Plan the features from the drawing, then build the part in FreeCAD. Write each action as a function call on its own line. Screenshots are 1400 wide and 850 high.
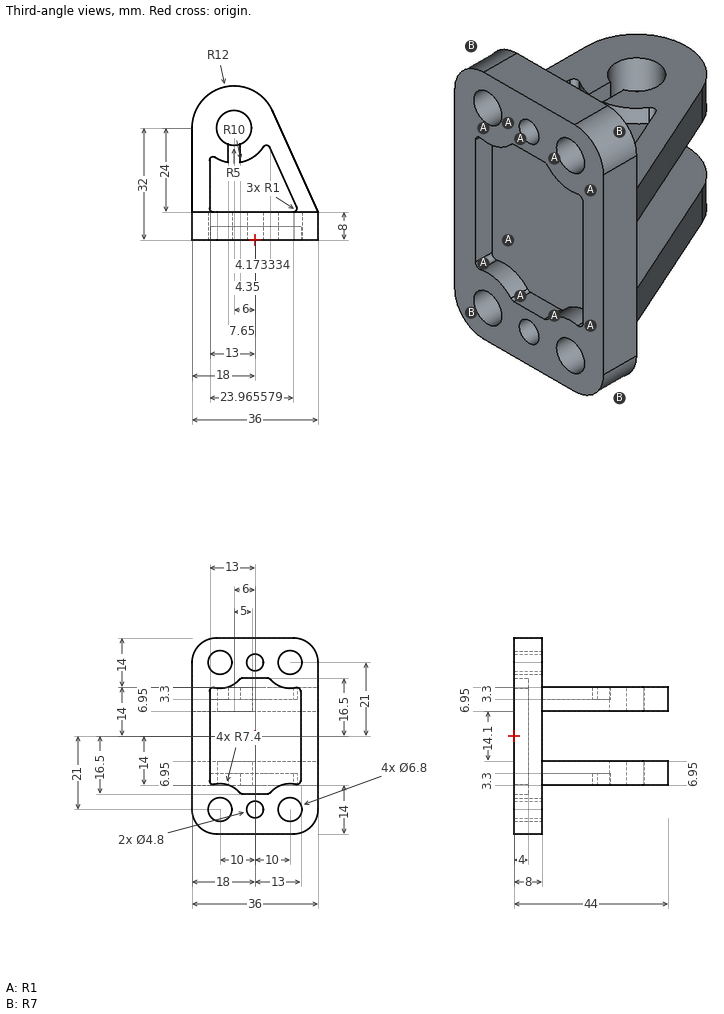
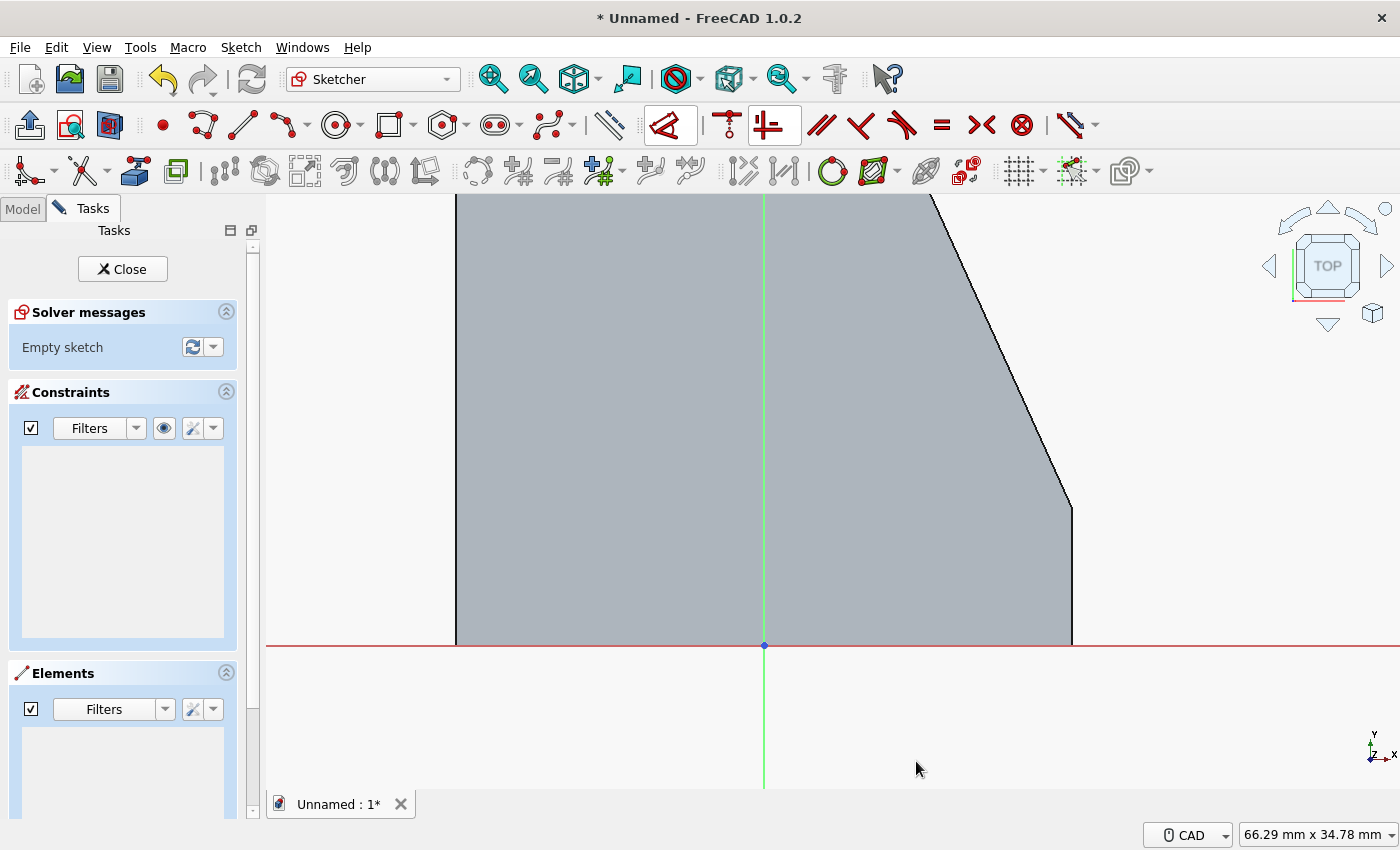
click(390, 126)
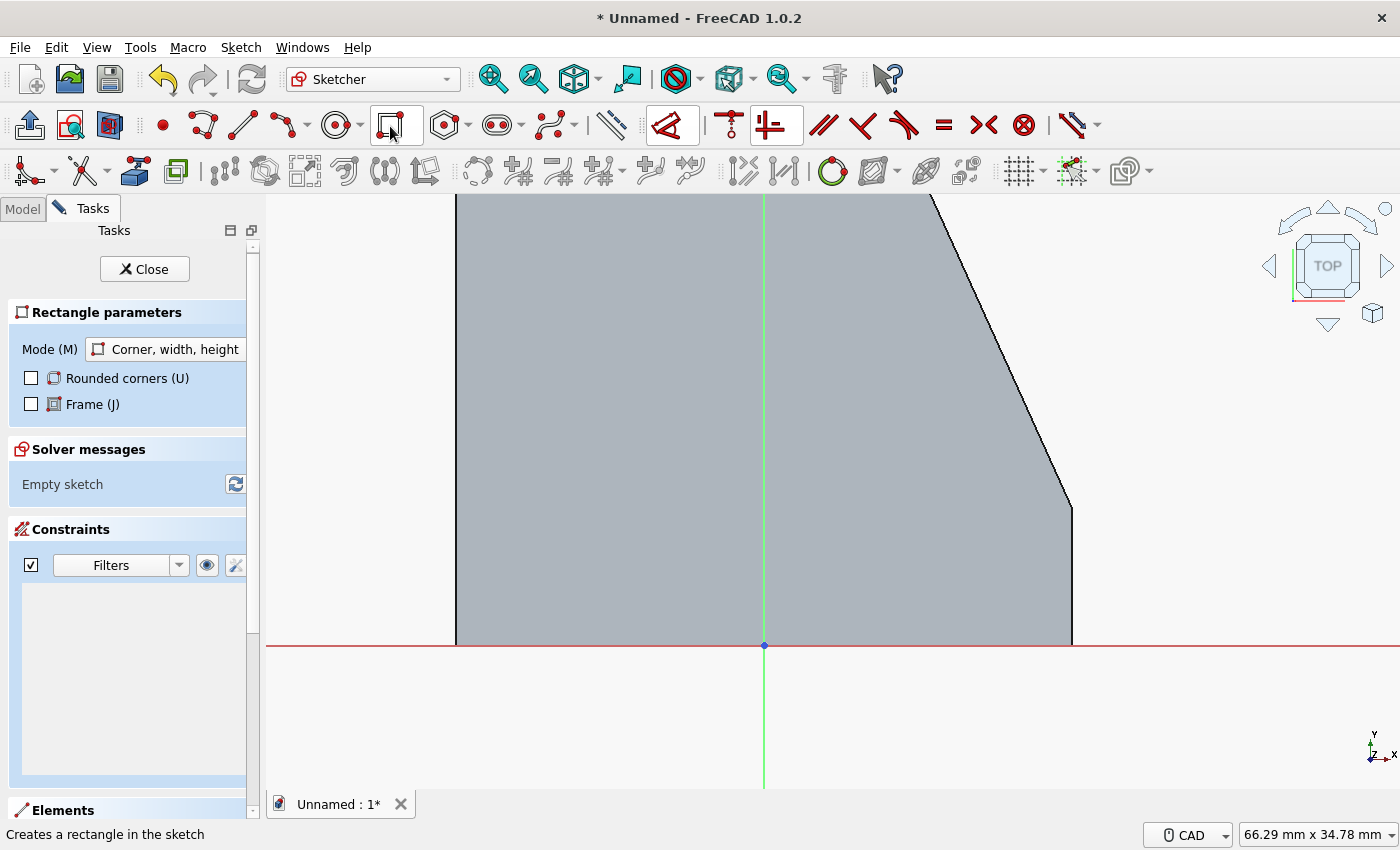
click(456, 509)
click(1072, 646)
key(Escape)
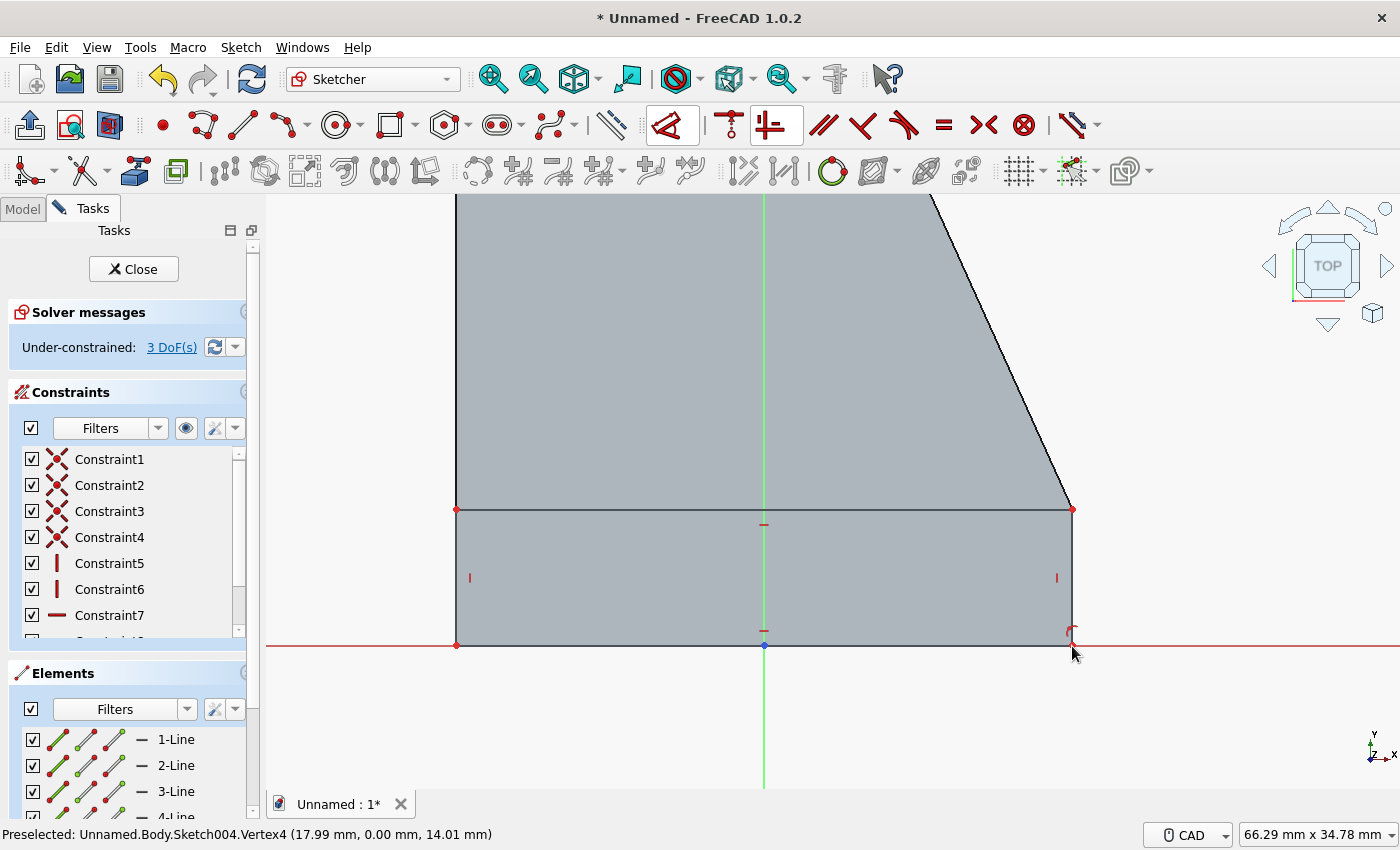
click(456, 551)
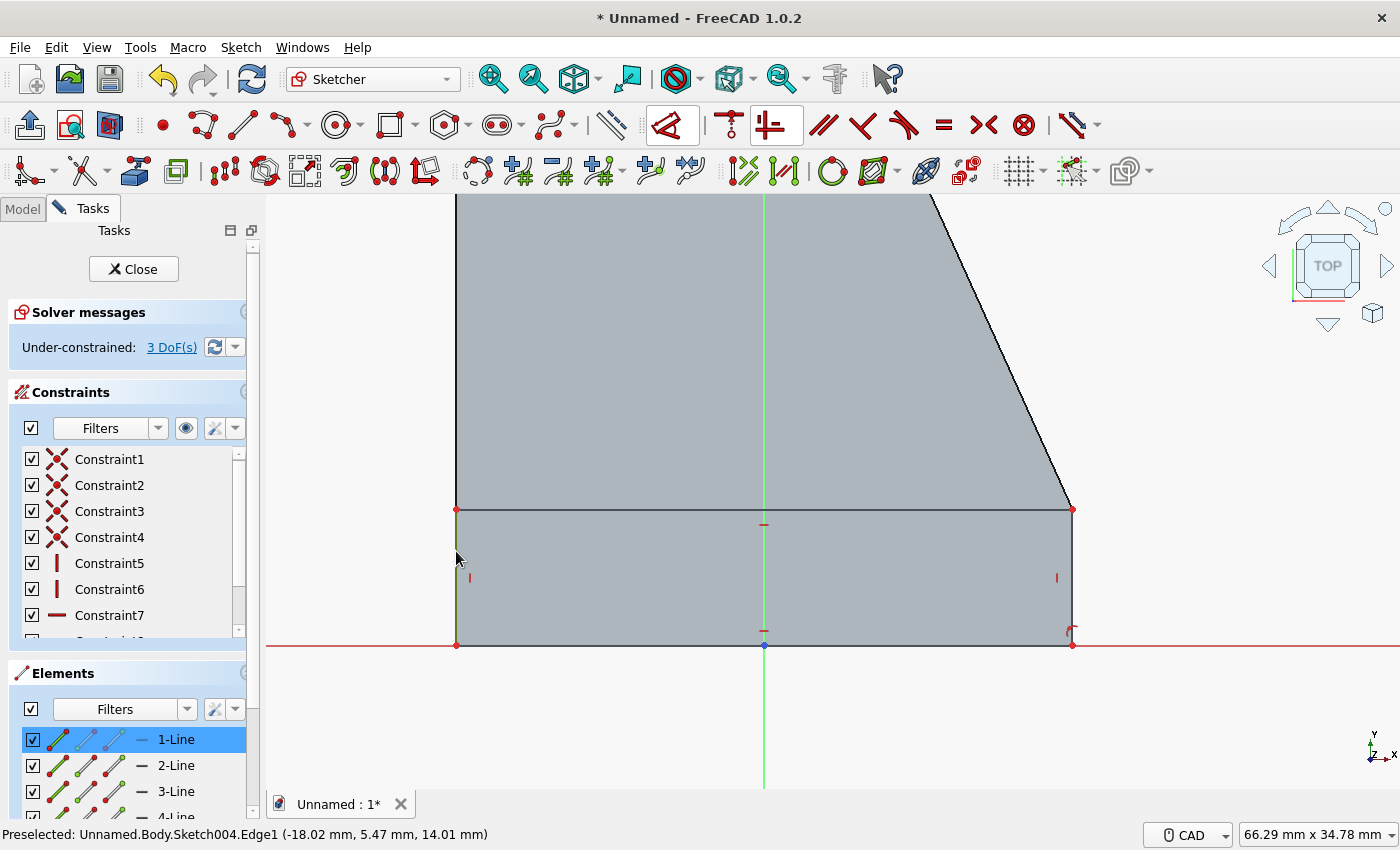
key(i)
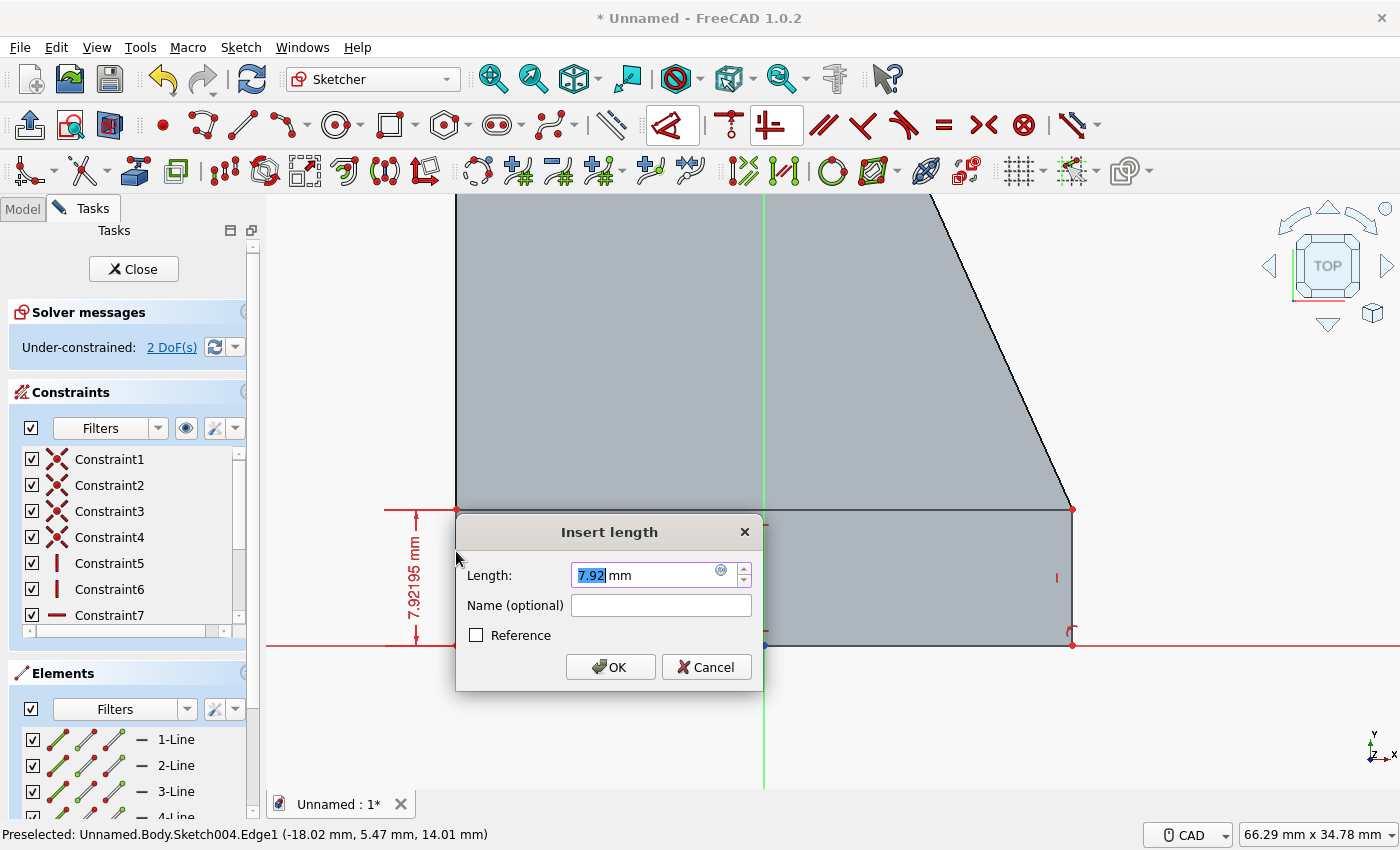
text(8)
key(Return)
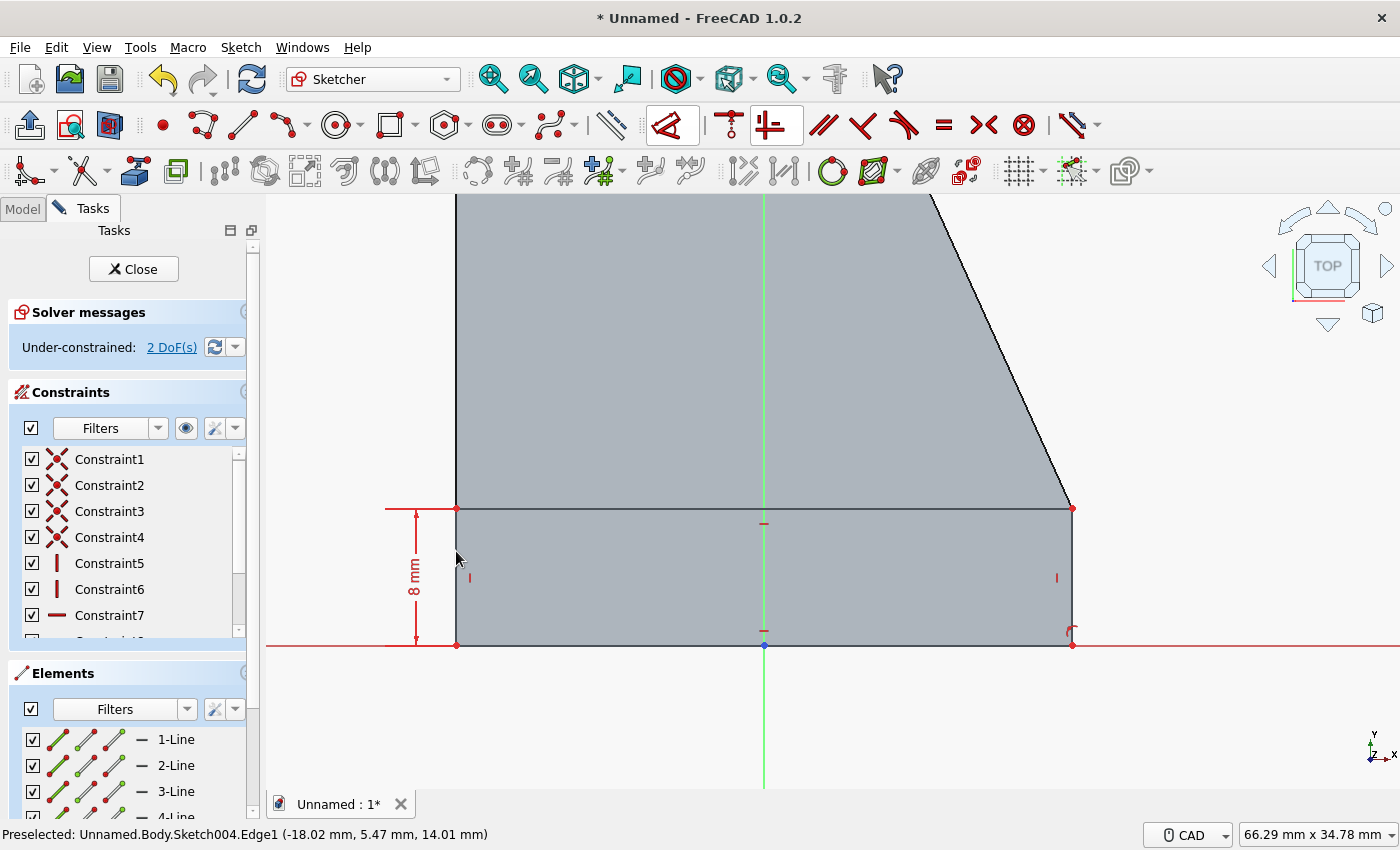
click(641, 646)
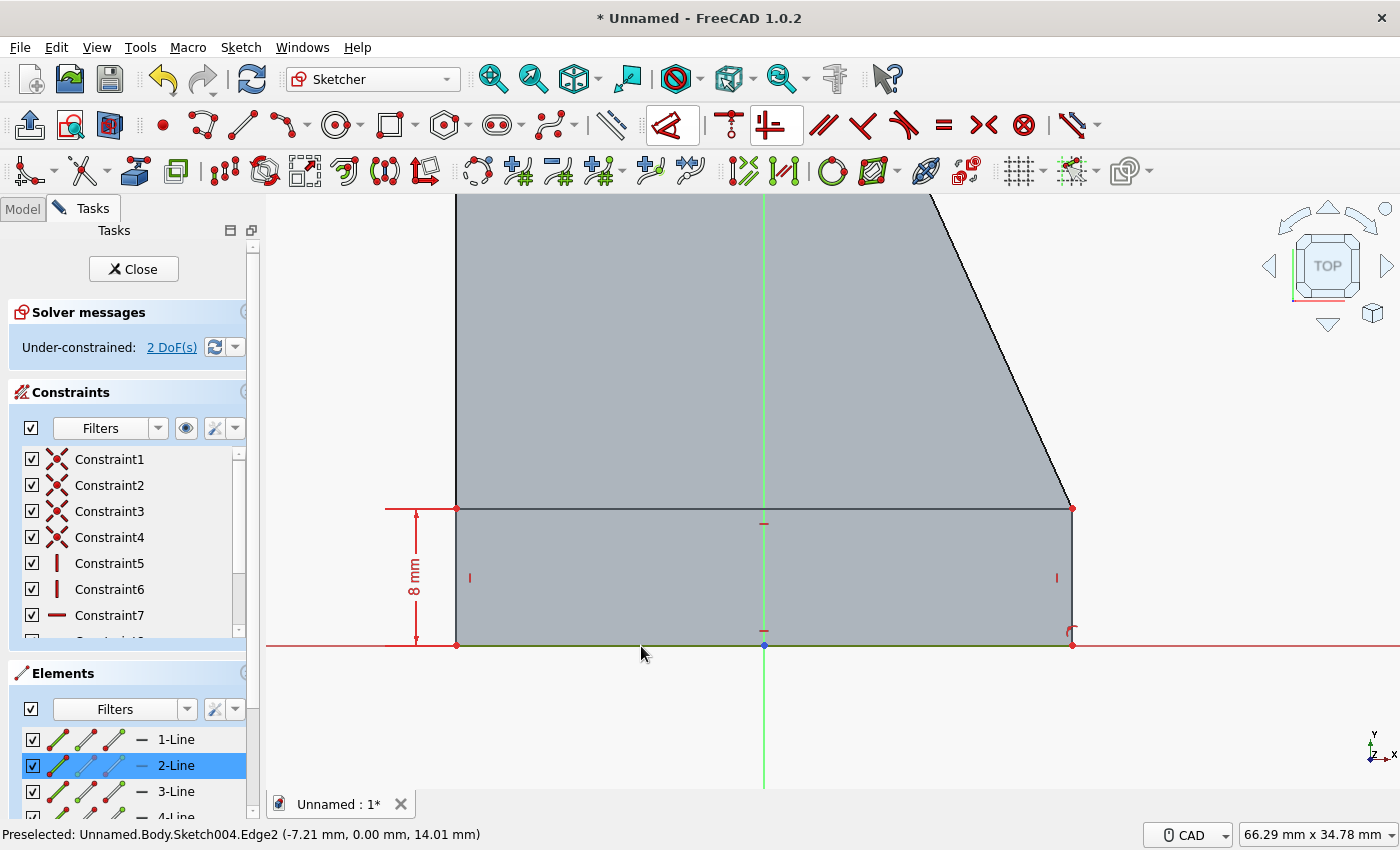
key(l)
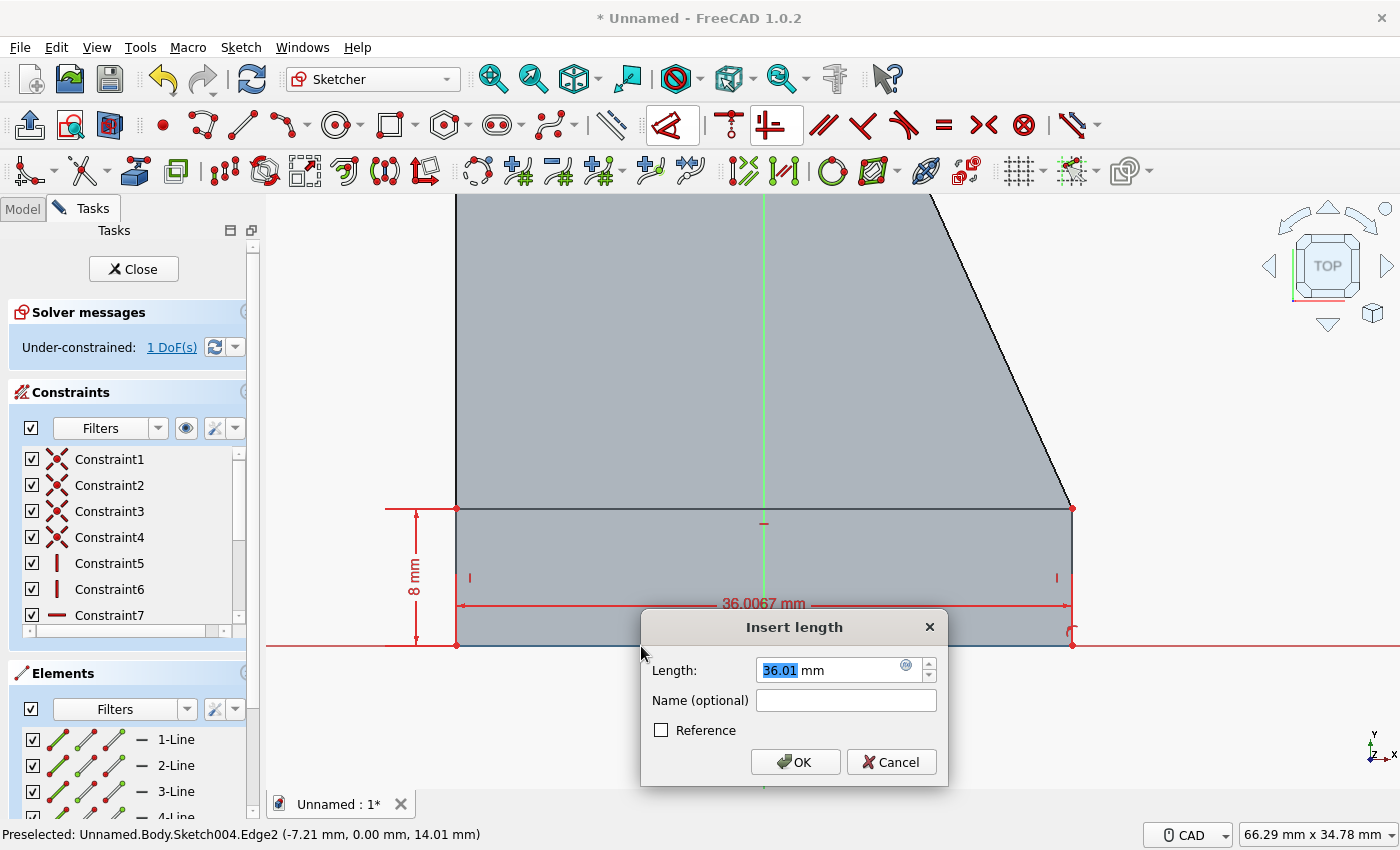
text(36)
key(Return)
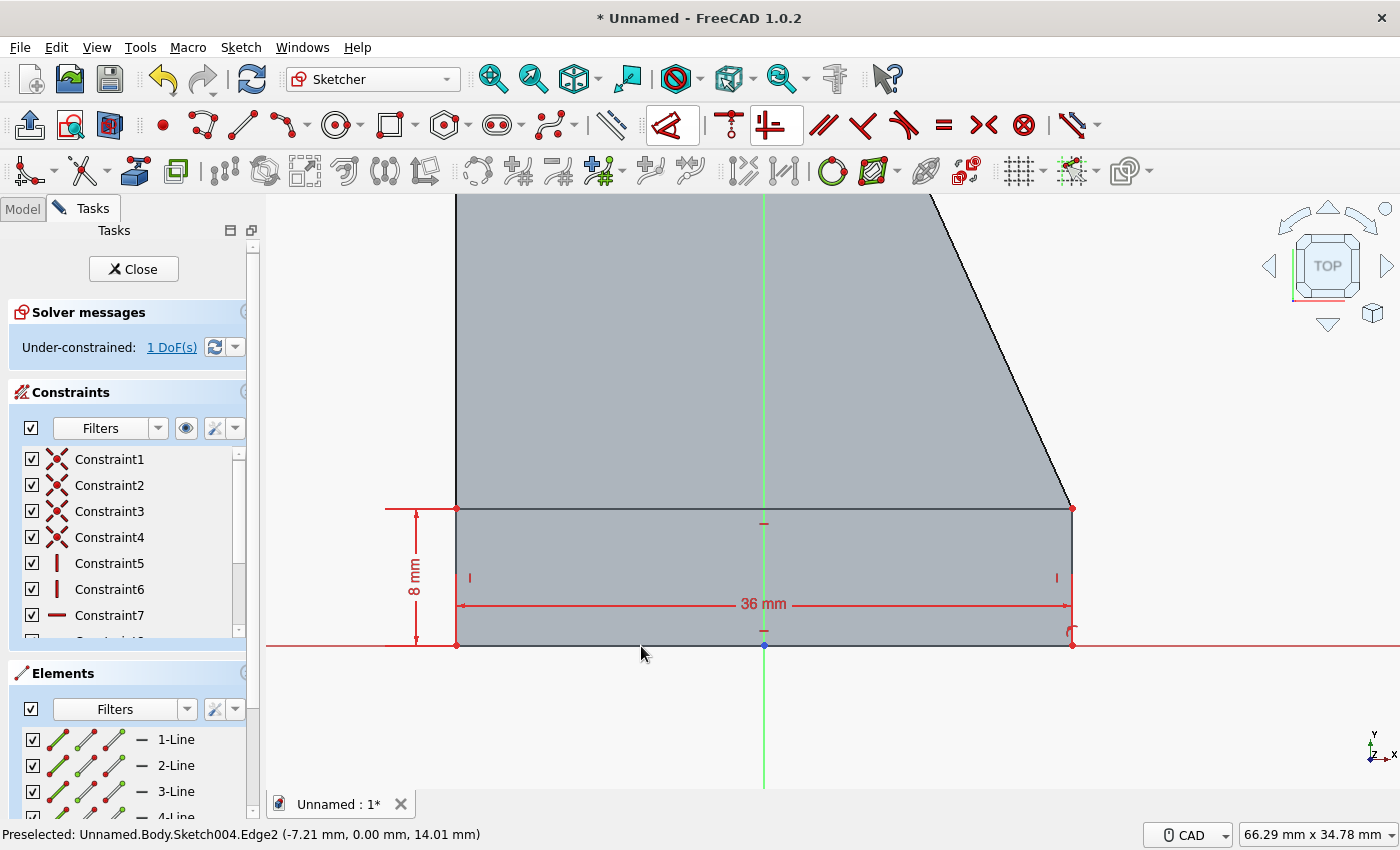
click(456, 509)